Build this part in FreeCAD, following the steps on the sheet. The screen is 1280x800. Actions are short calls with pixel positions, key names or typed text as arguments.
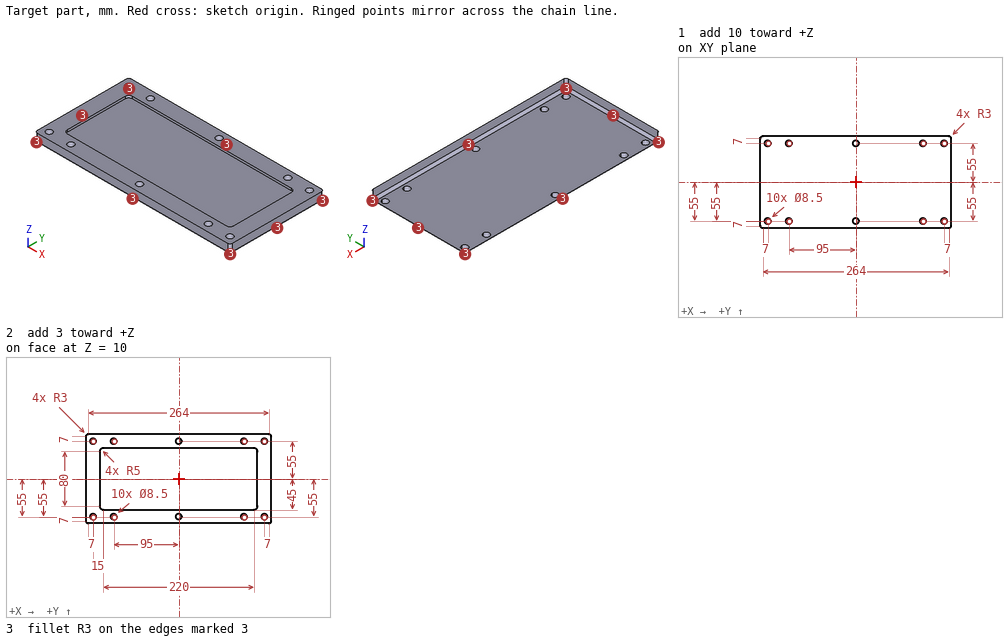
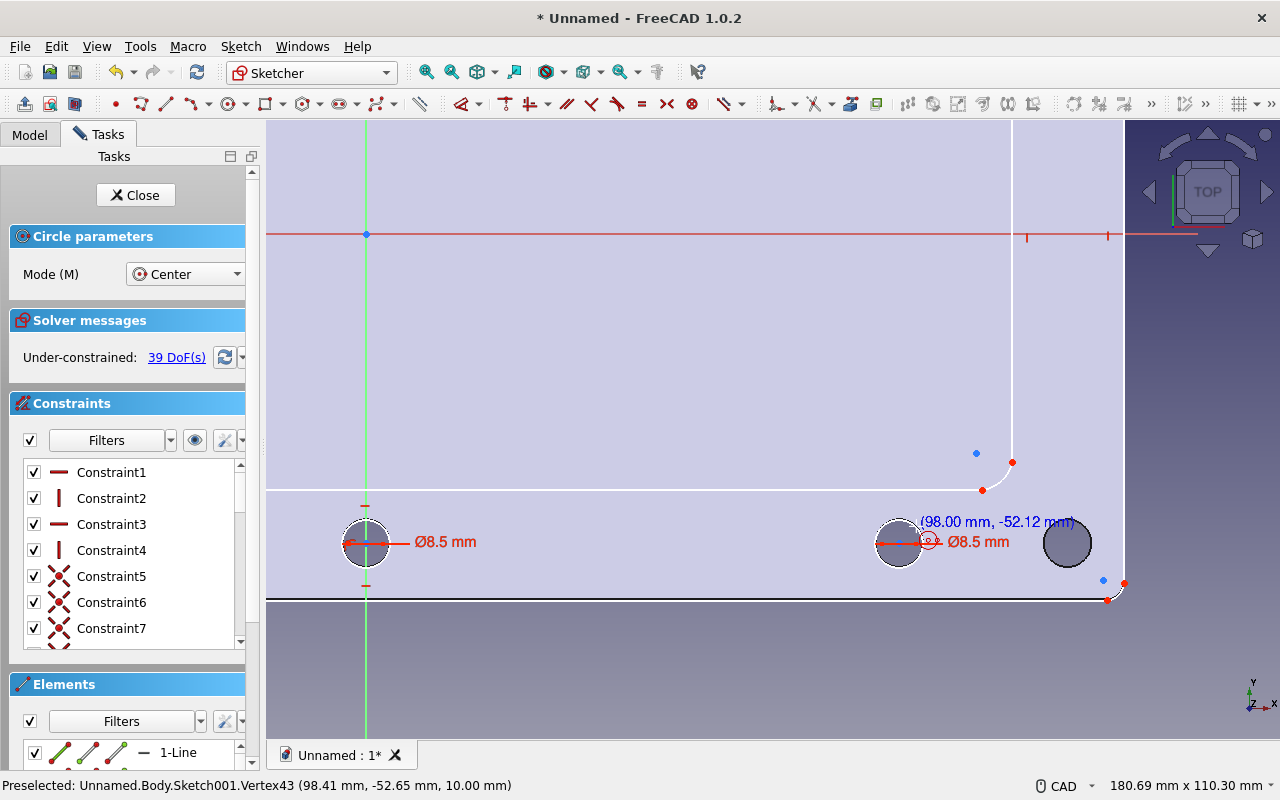
click(1068, 543)
move(1084, 526)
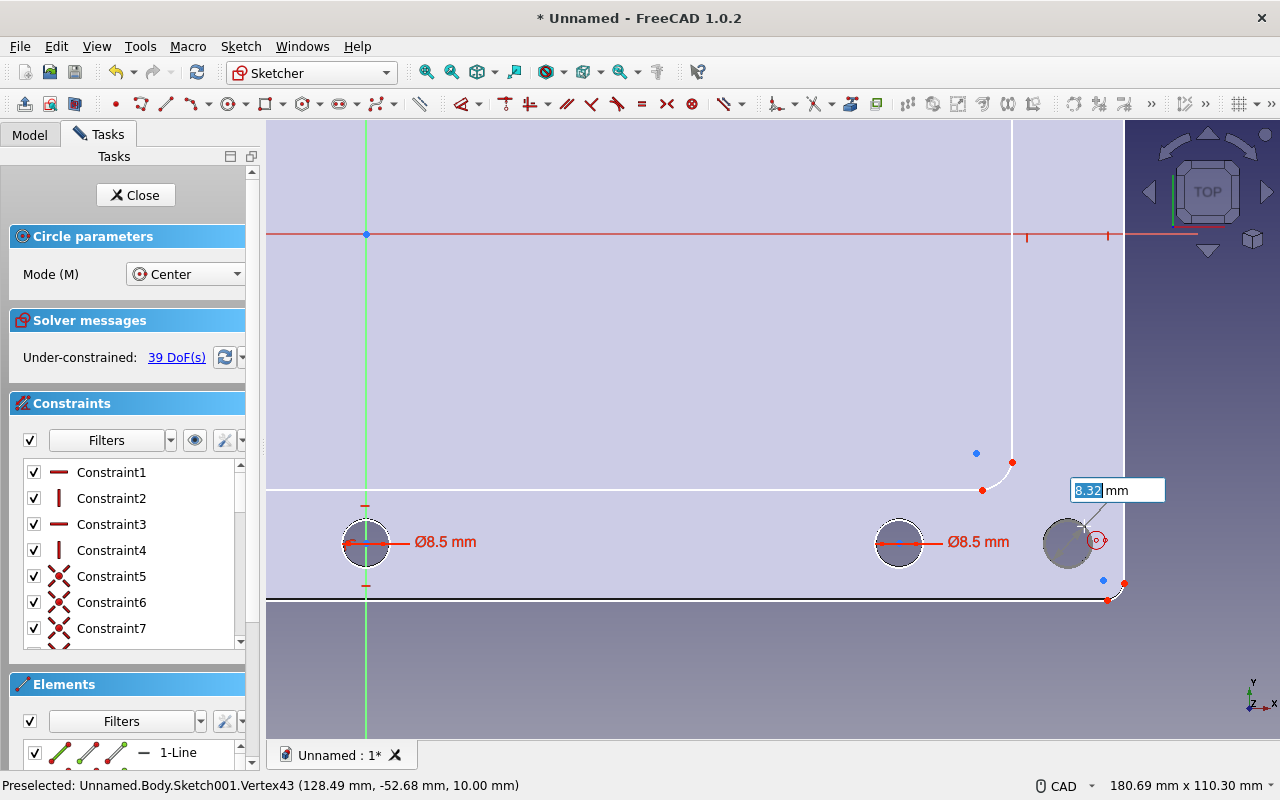
text(8.5)
key(Return)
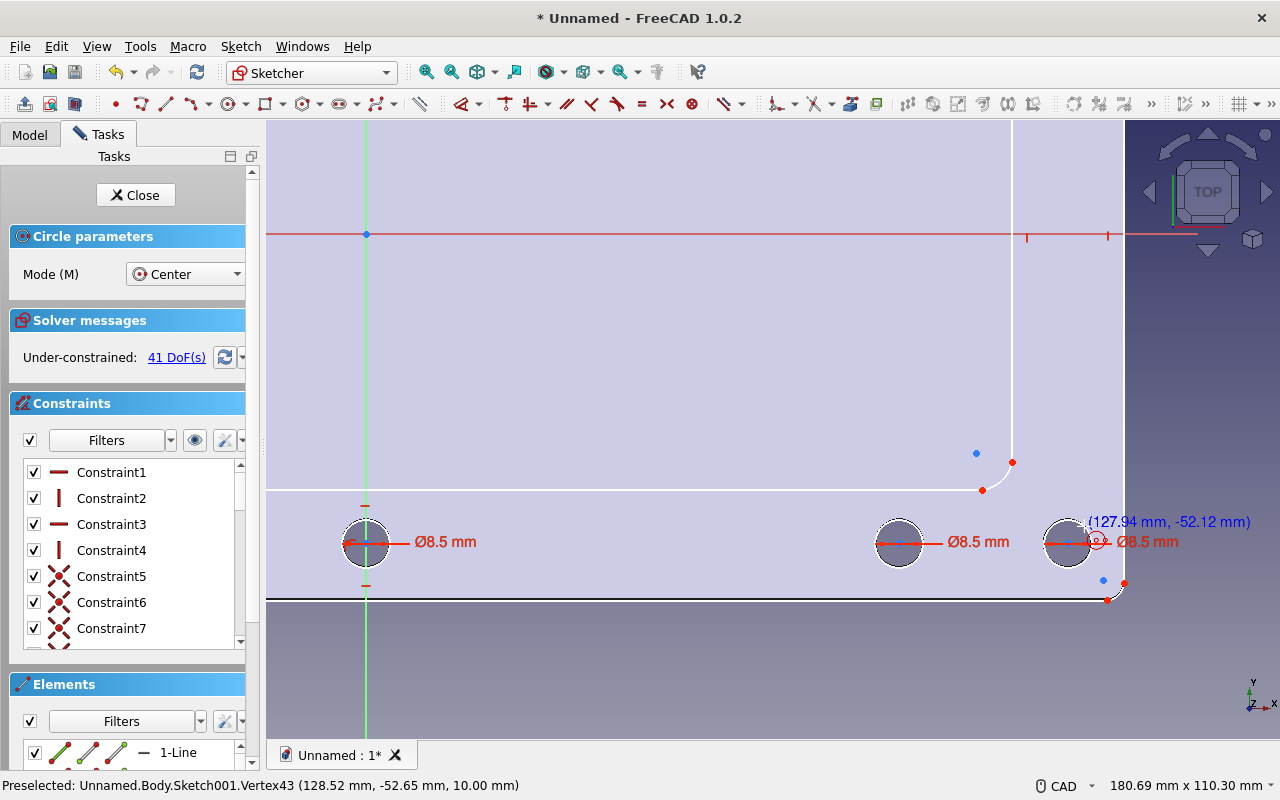
scroll(901, 543, down, 5)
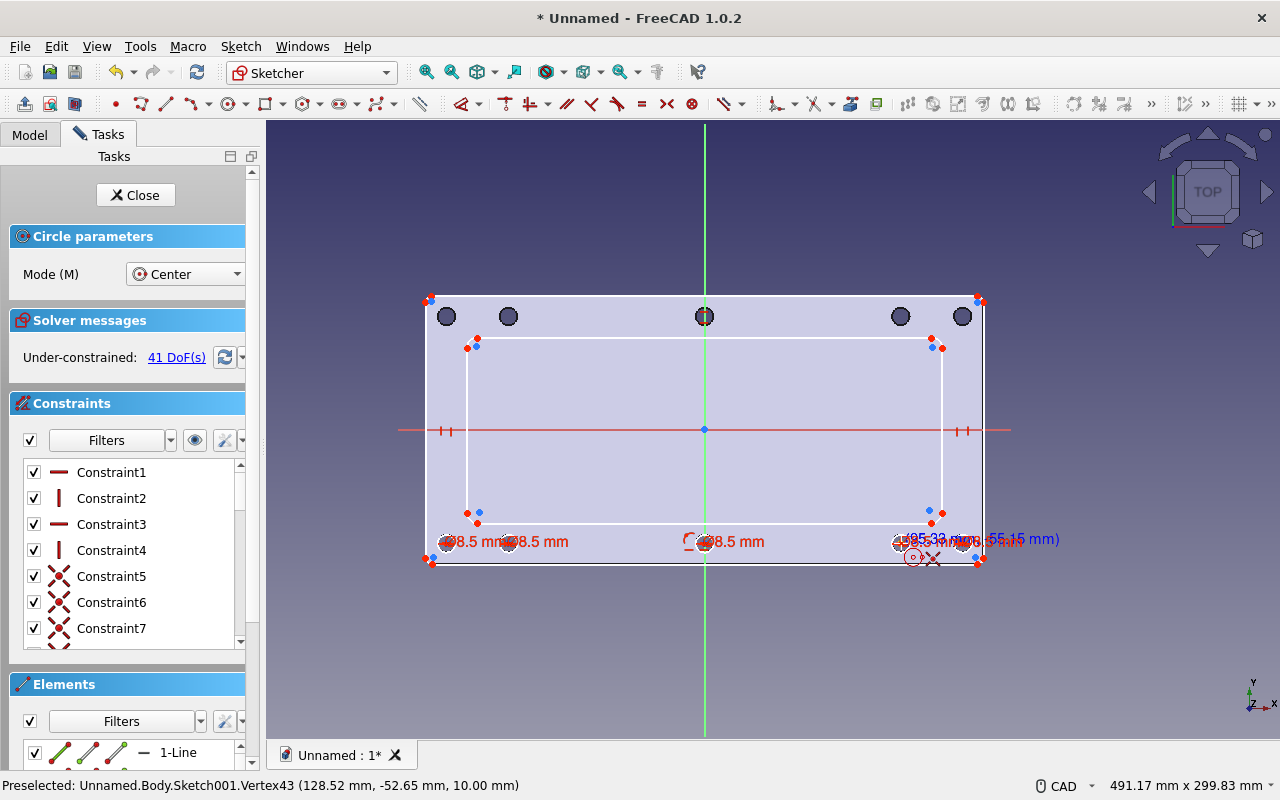
scroll(447, 316, up, 5)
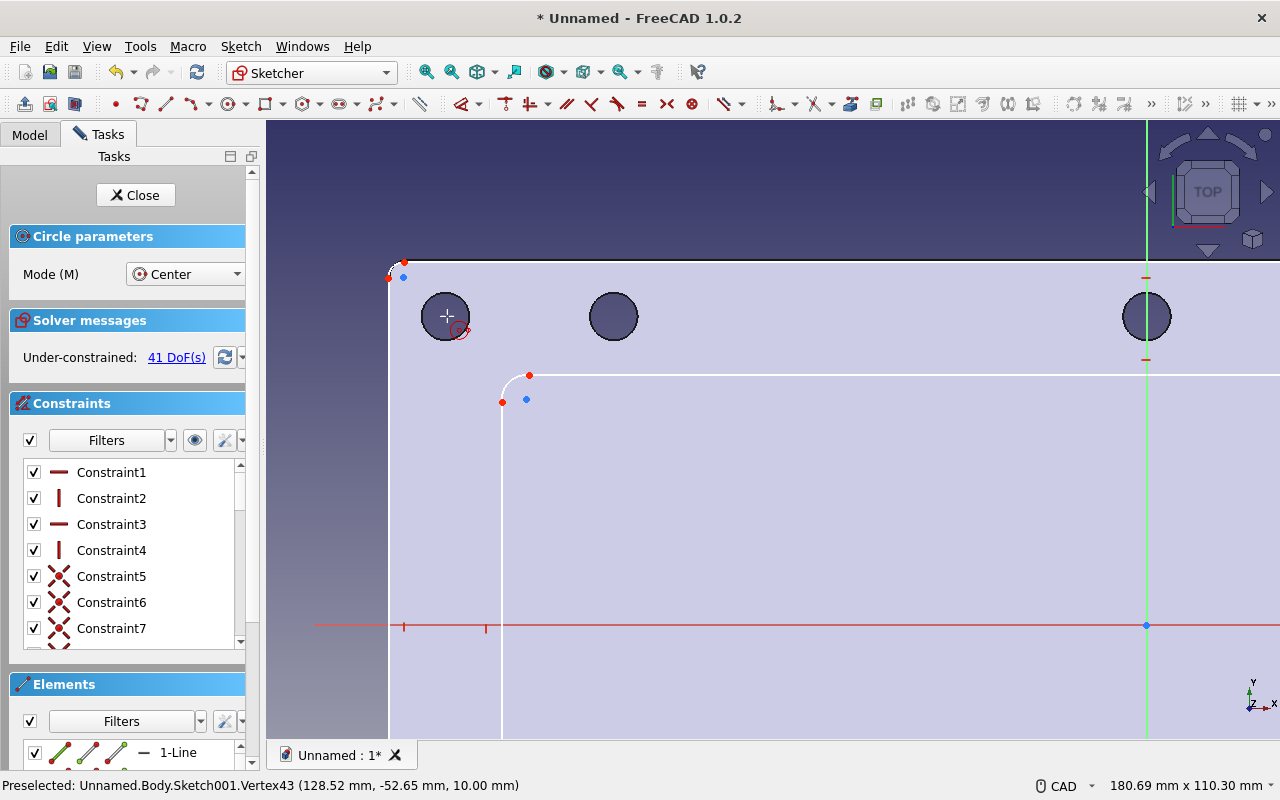
click(445, 317)
move(462, 300)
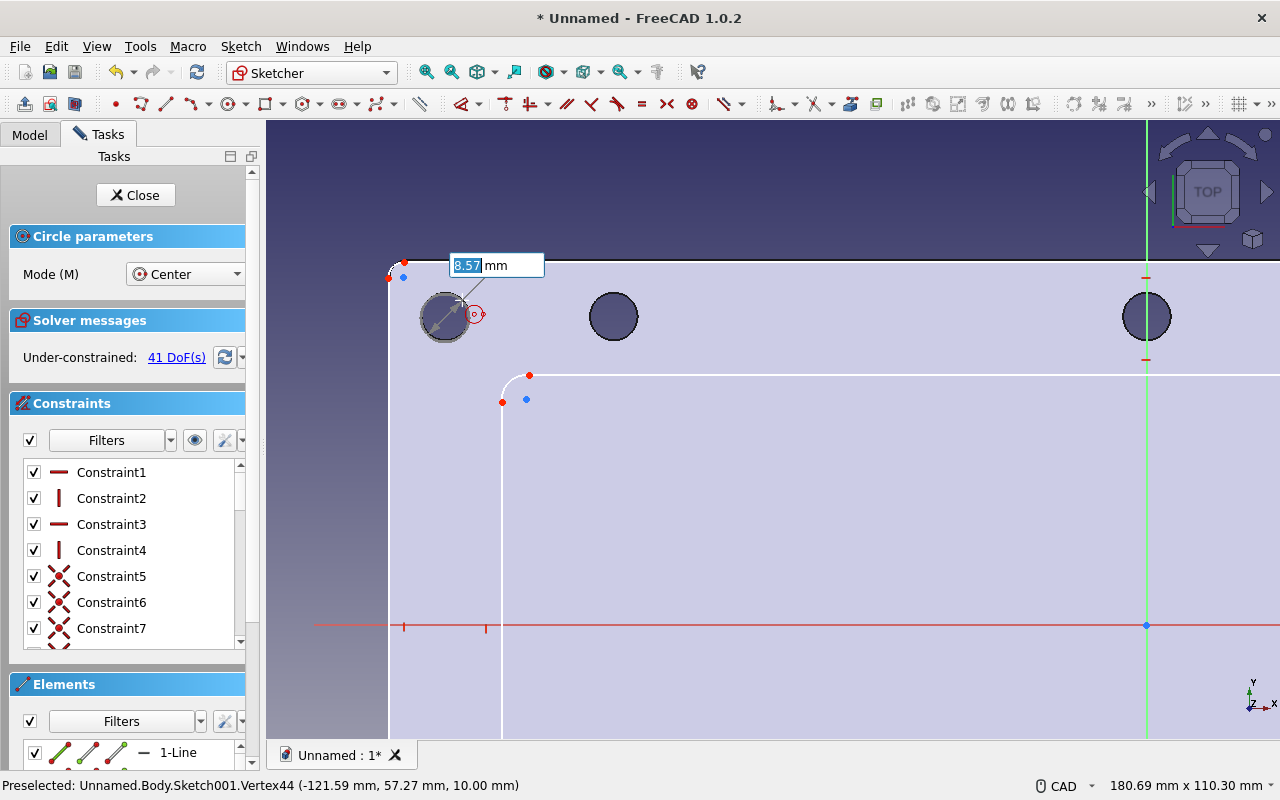
text(8.5)
key(Return)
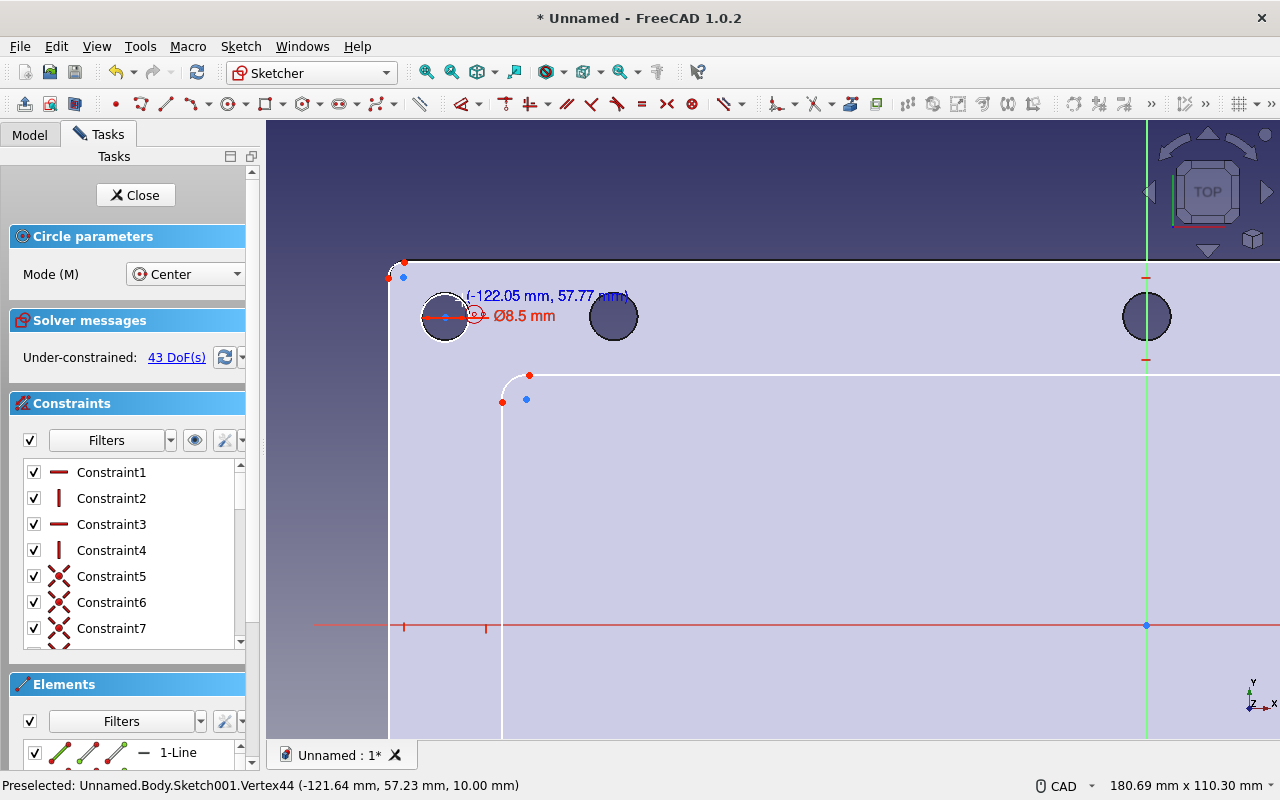
click(614, 317)
move(631, 300)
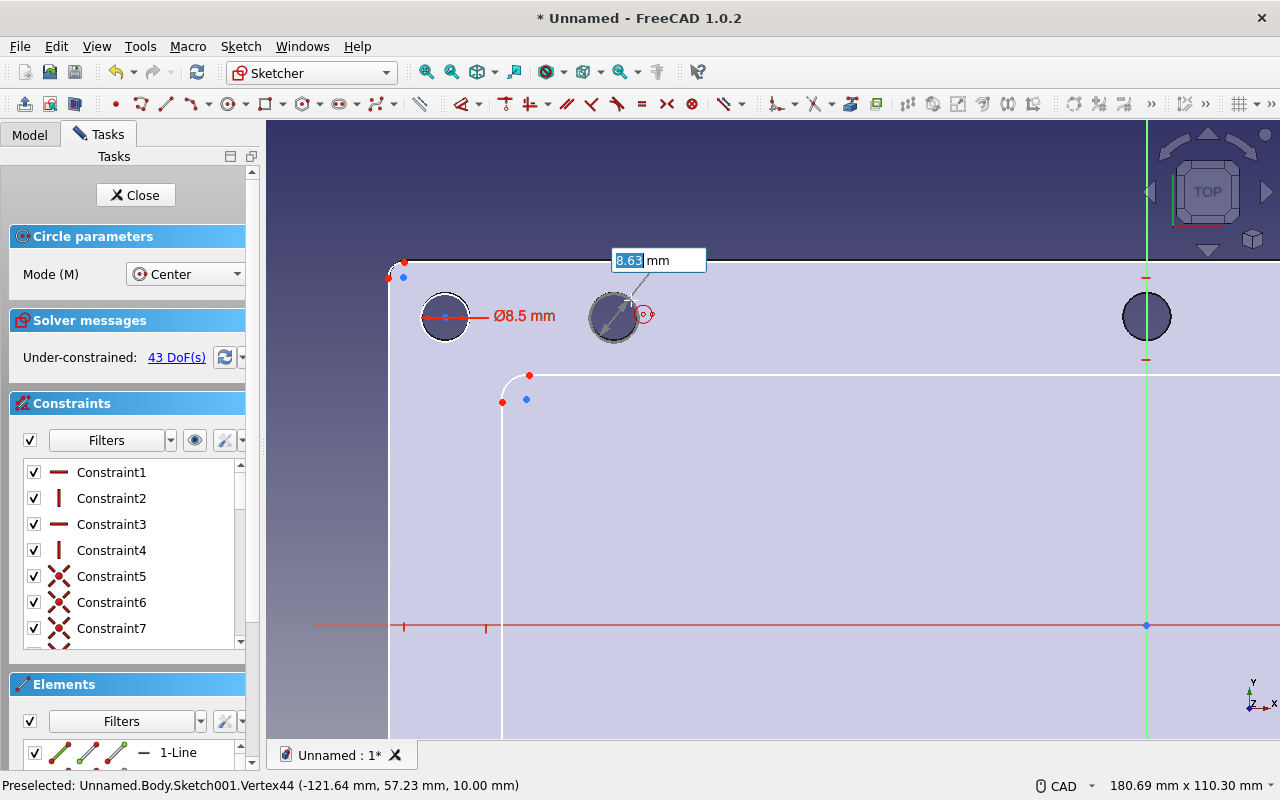
text(8.5)
key(Return)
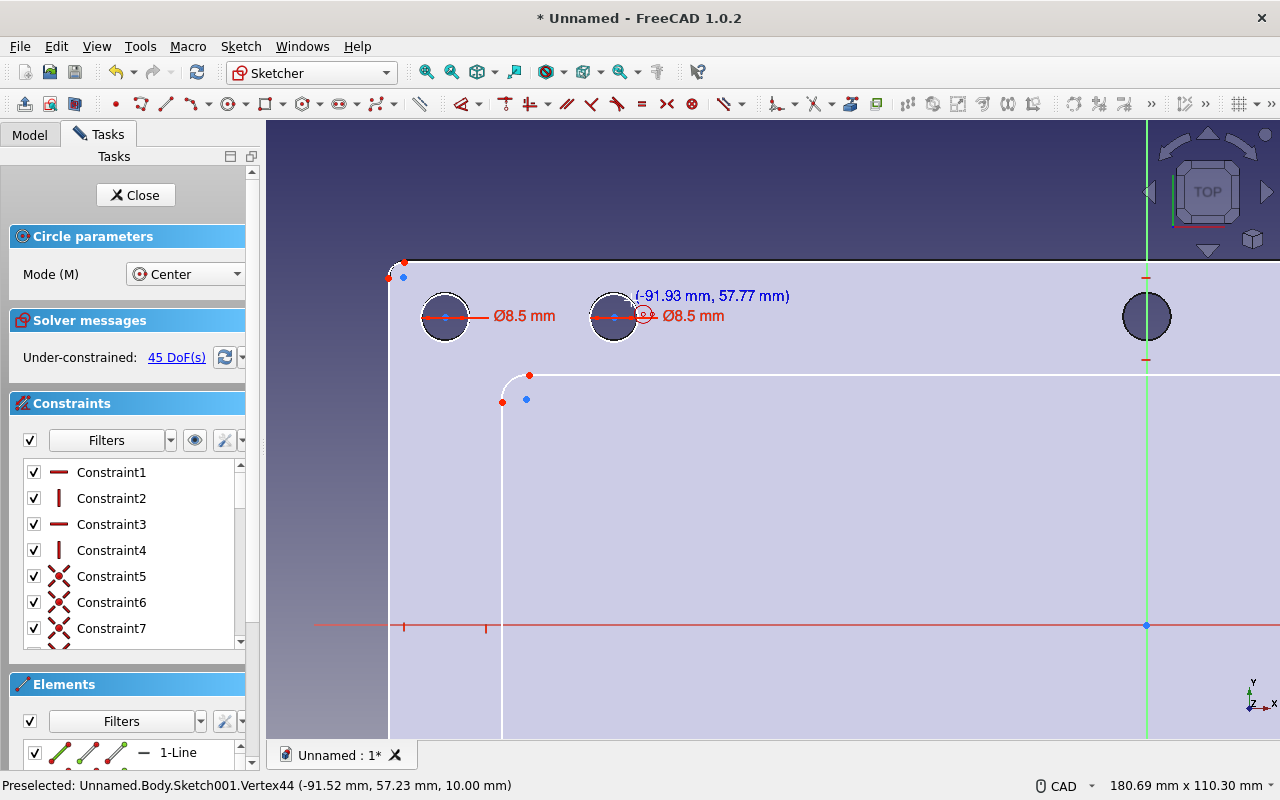
scroll(447, 316, down, 5)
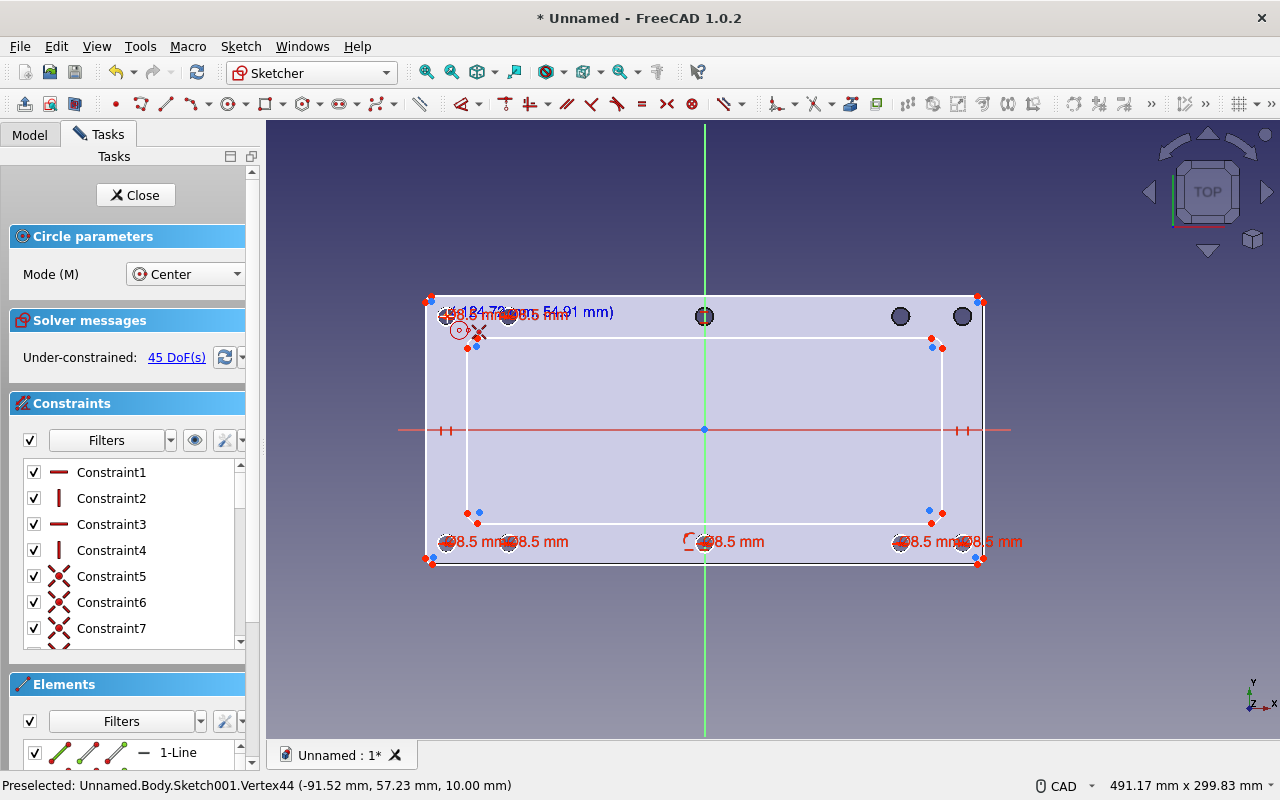
scroll(705, 316, up, 5)